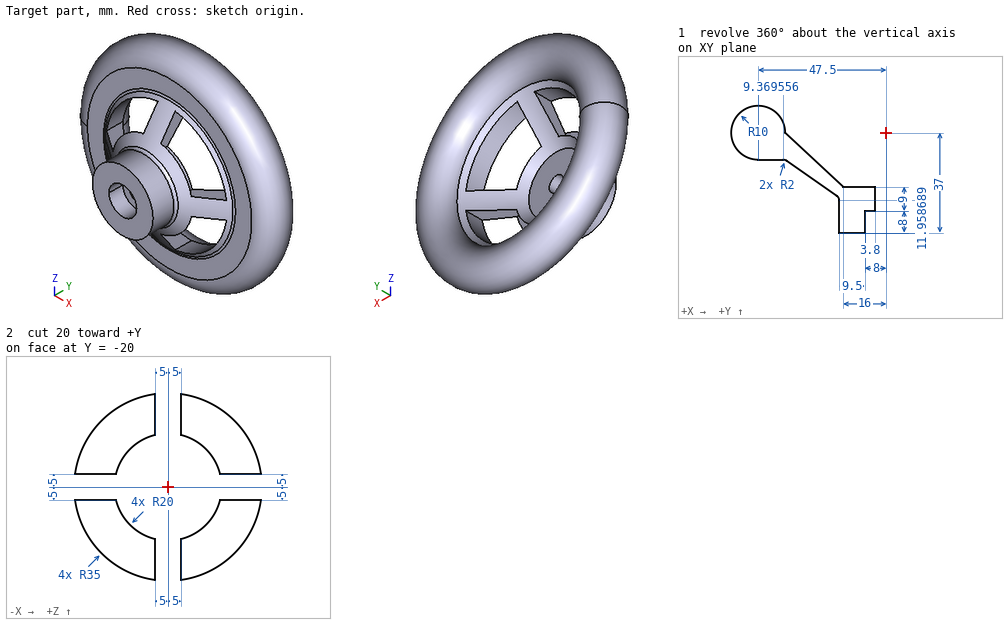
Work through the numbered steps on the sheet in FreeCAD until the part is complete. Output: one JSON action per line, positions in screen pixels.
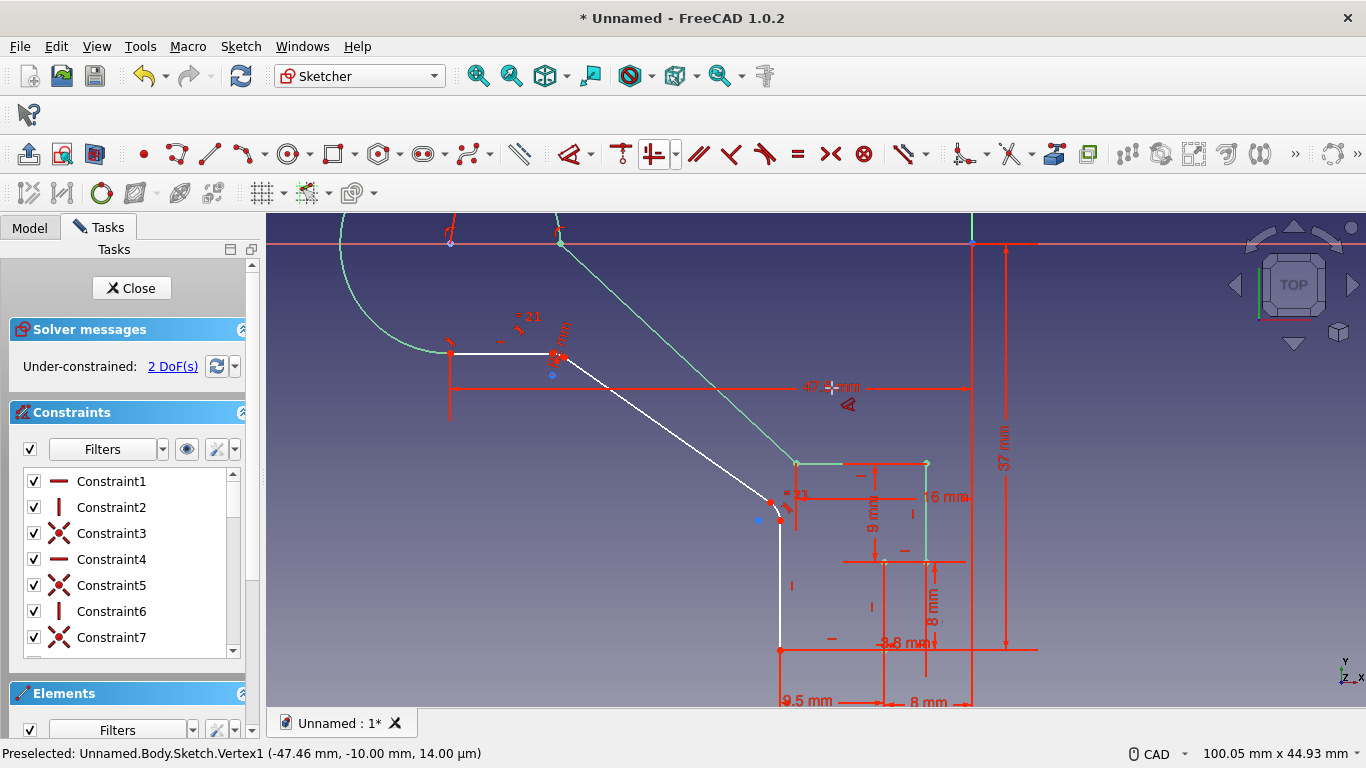
{"action": "left_click", "coordinate": [481, 354]}
{"action": "left_click", "coordinate": [501, 320]}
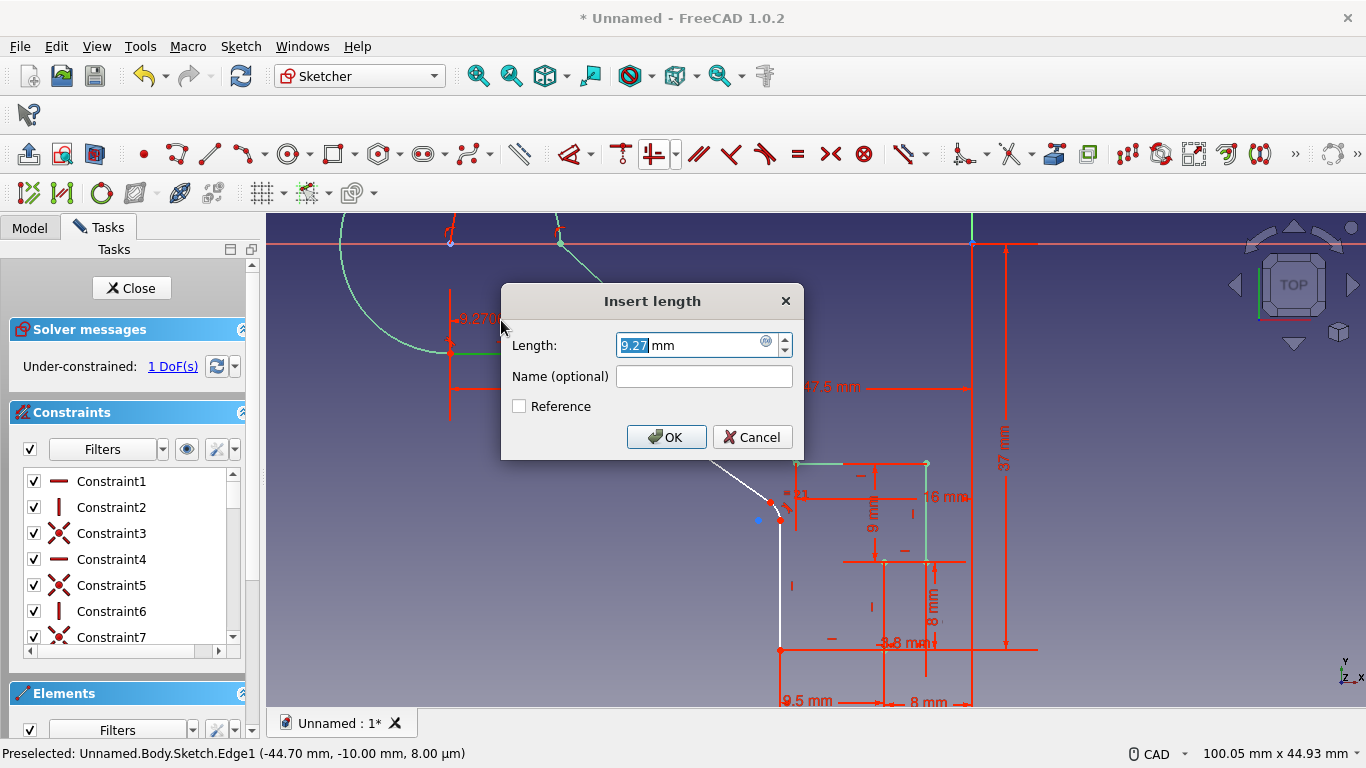
{"action": "type", "text": "9.369556"}
{"action": "key", "text": "Return"}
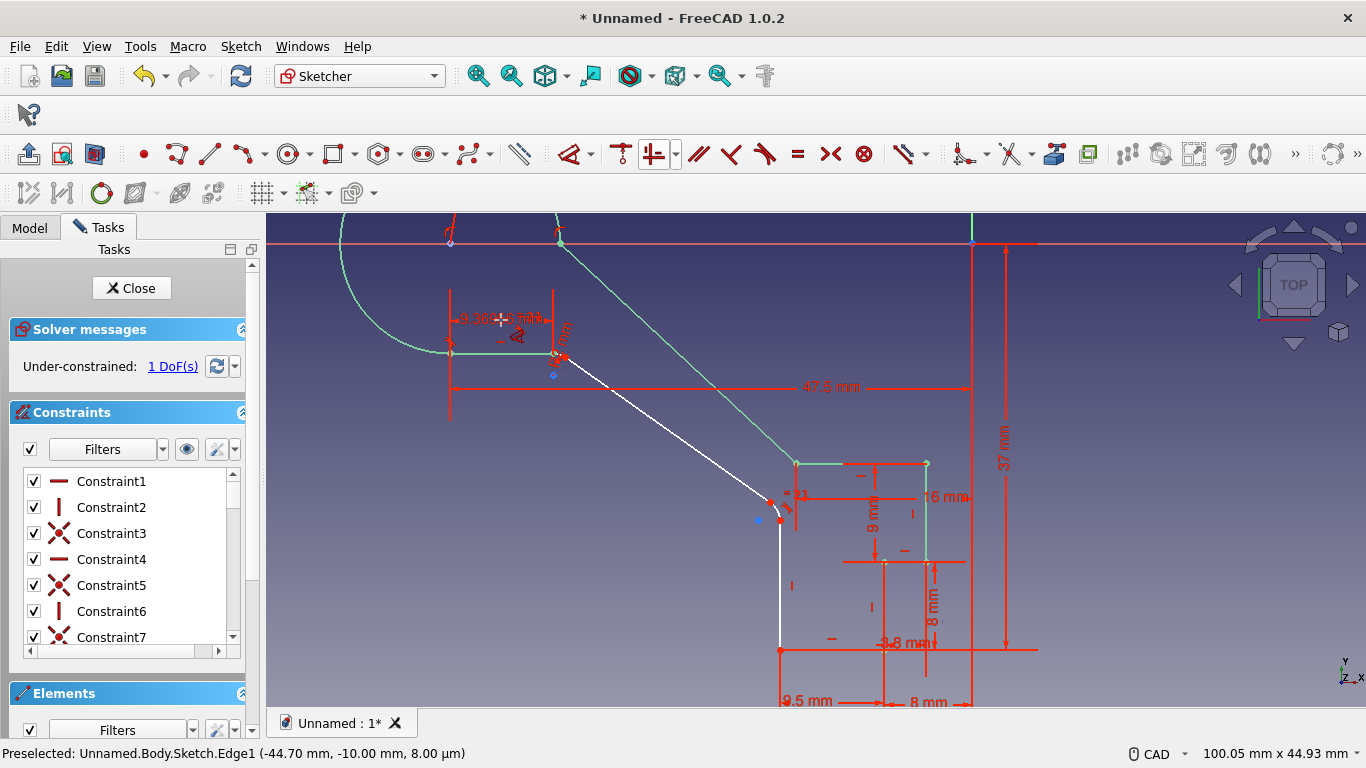
{"action": "left_click", "coordinate": [780, 560]}
{"action": "left_click", "coordinate": [814, 586]}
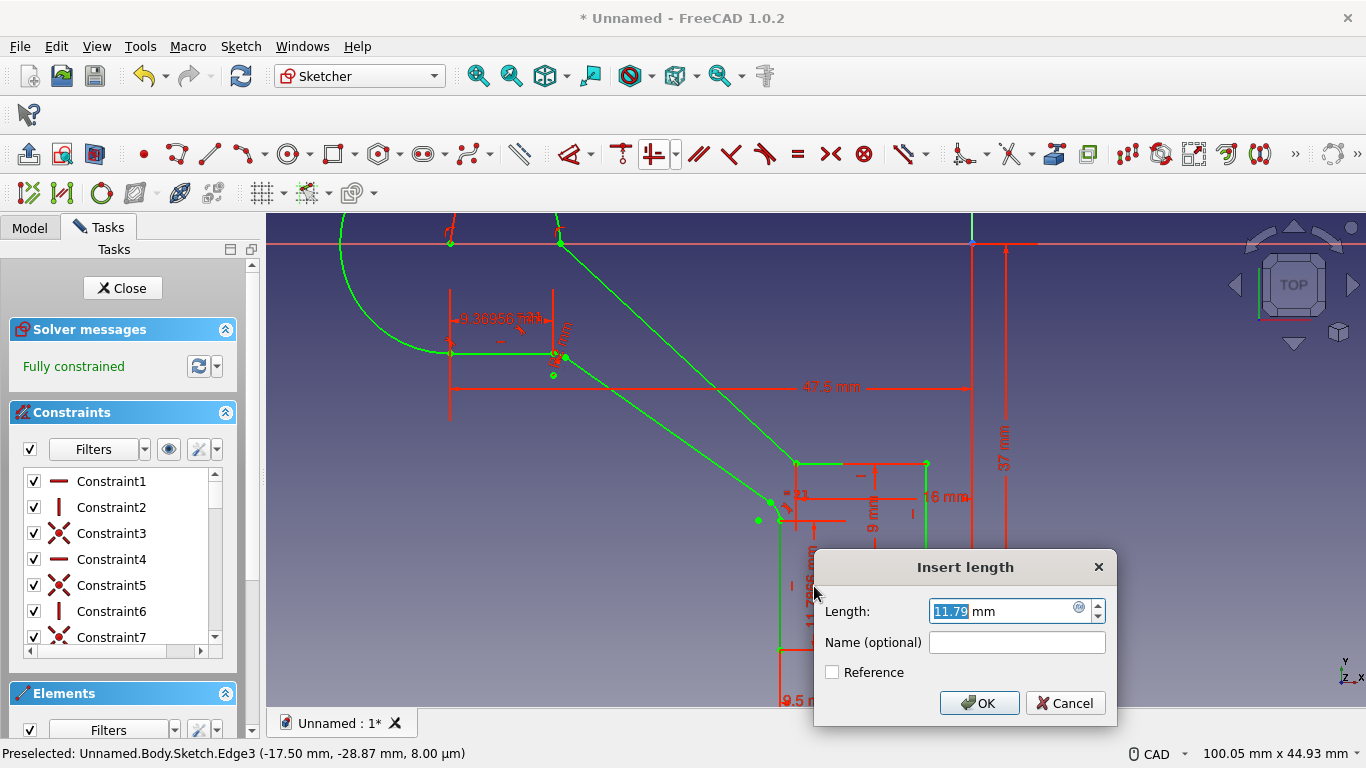
{"action": "type", "text": "11.958689"}
{"action": "key", "text": "Return"}
{"action": "key", "text": "Escape"}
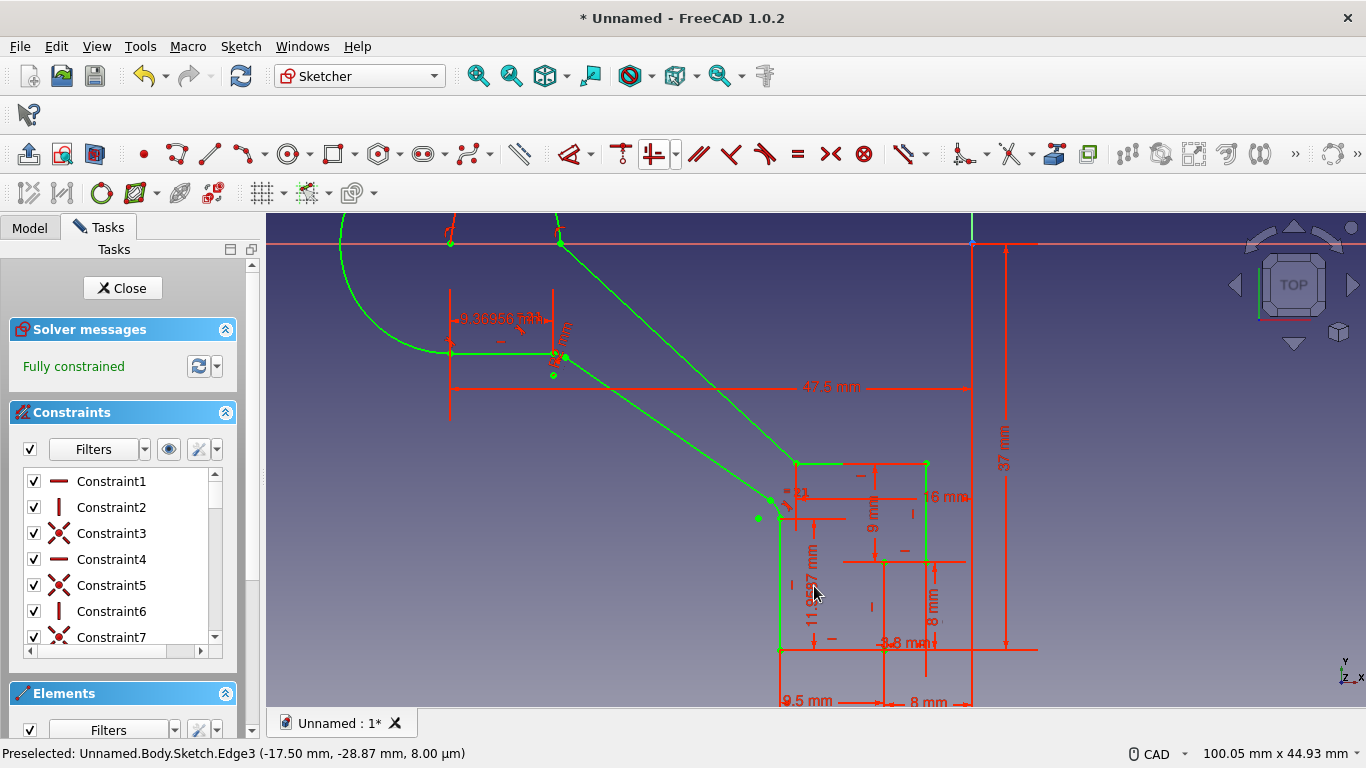
{"action": "left_click", "coordinate": [123, 288]}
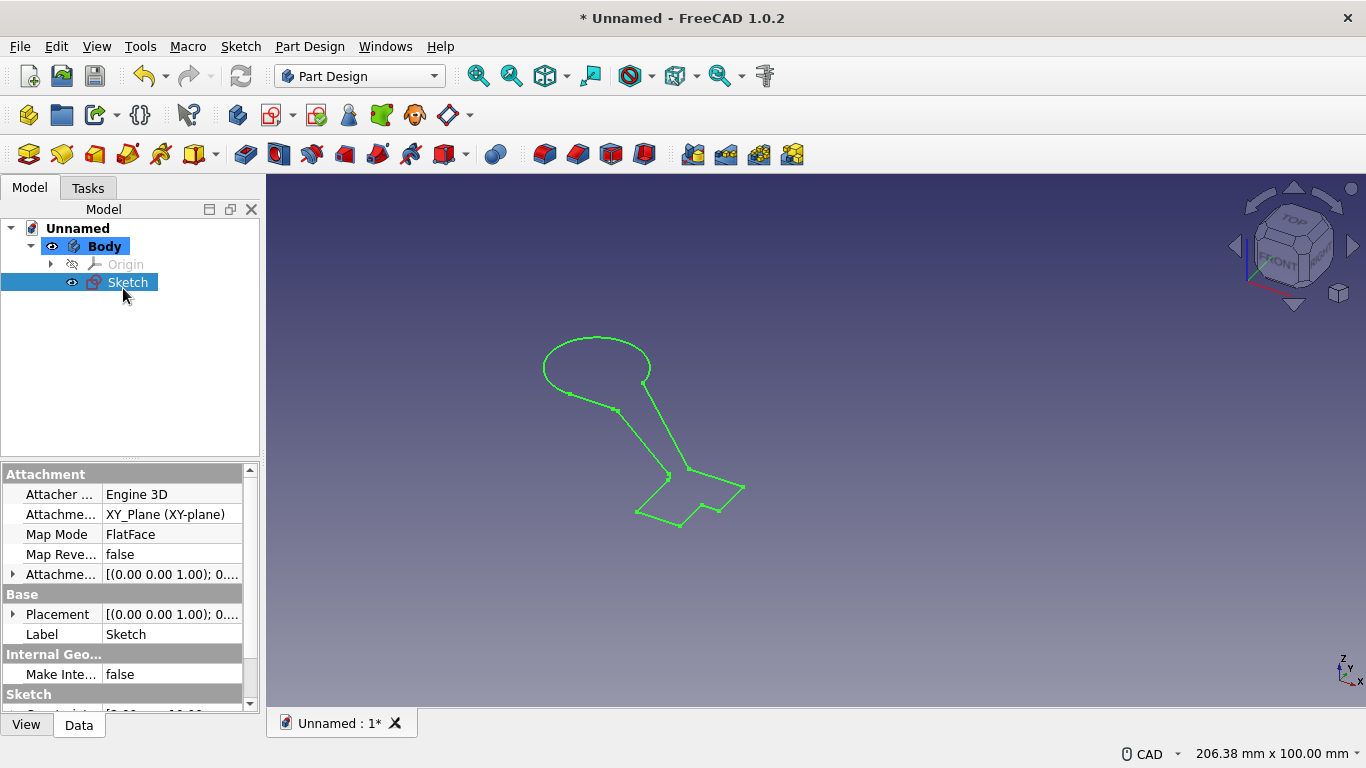
{"action": "left_click", "coordinate": [62, 154]}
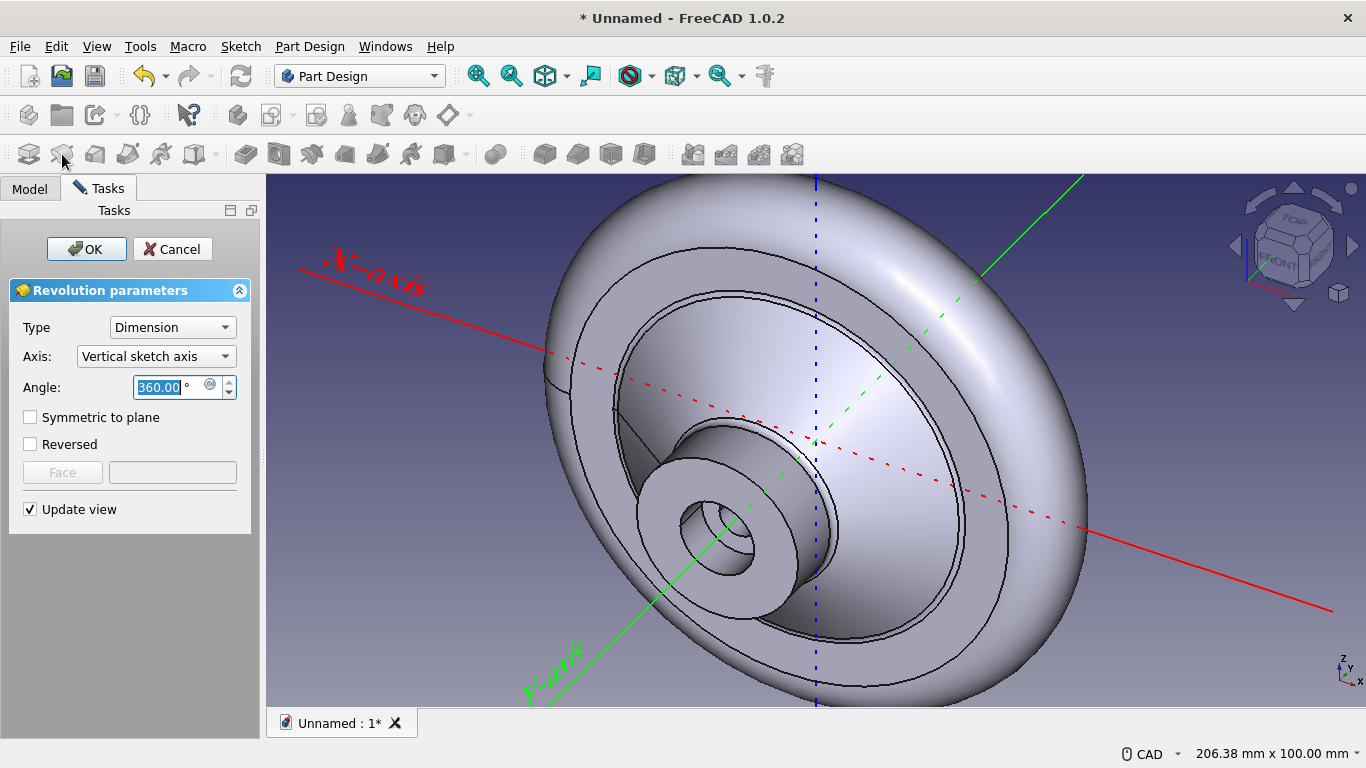
{"action": "left_click", "coordinate": [87, 249]}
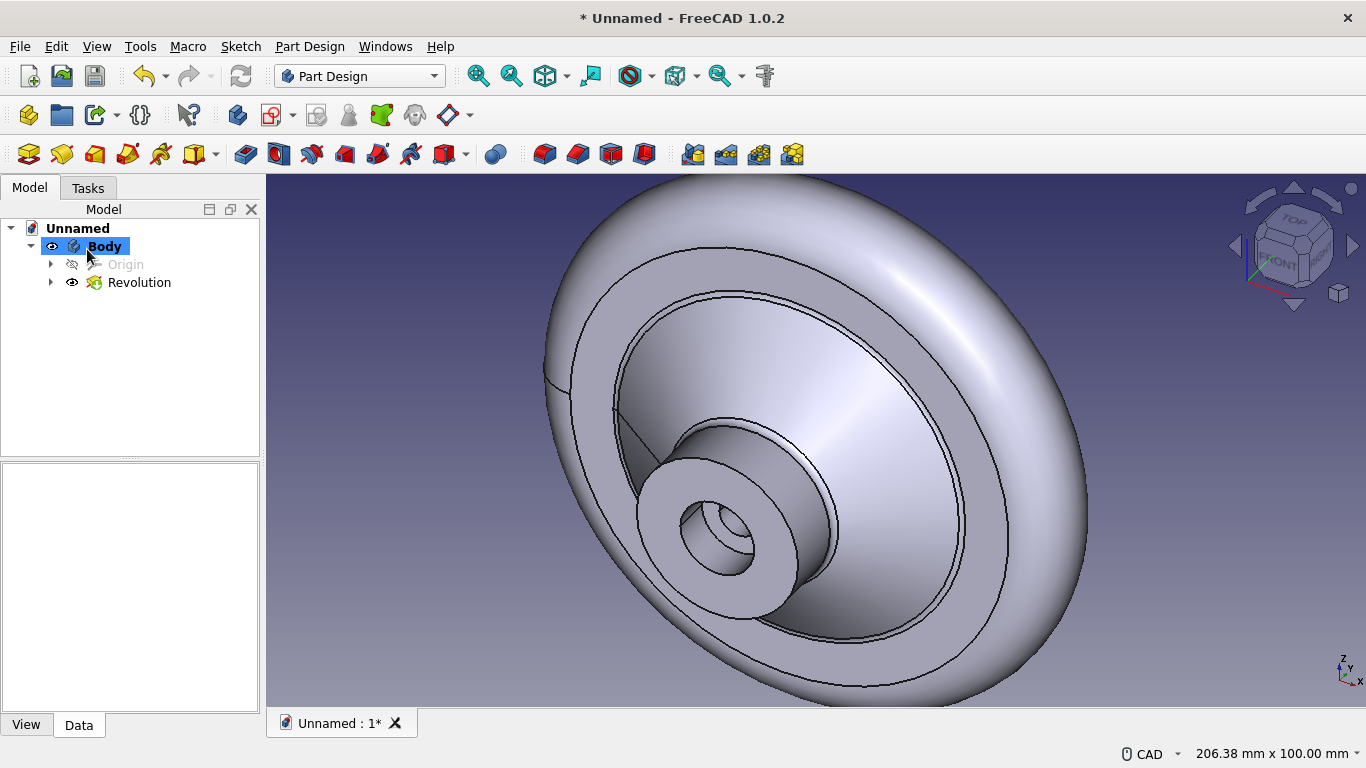
{"action": "key", "text": "v f"}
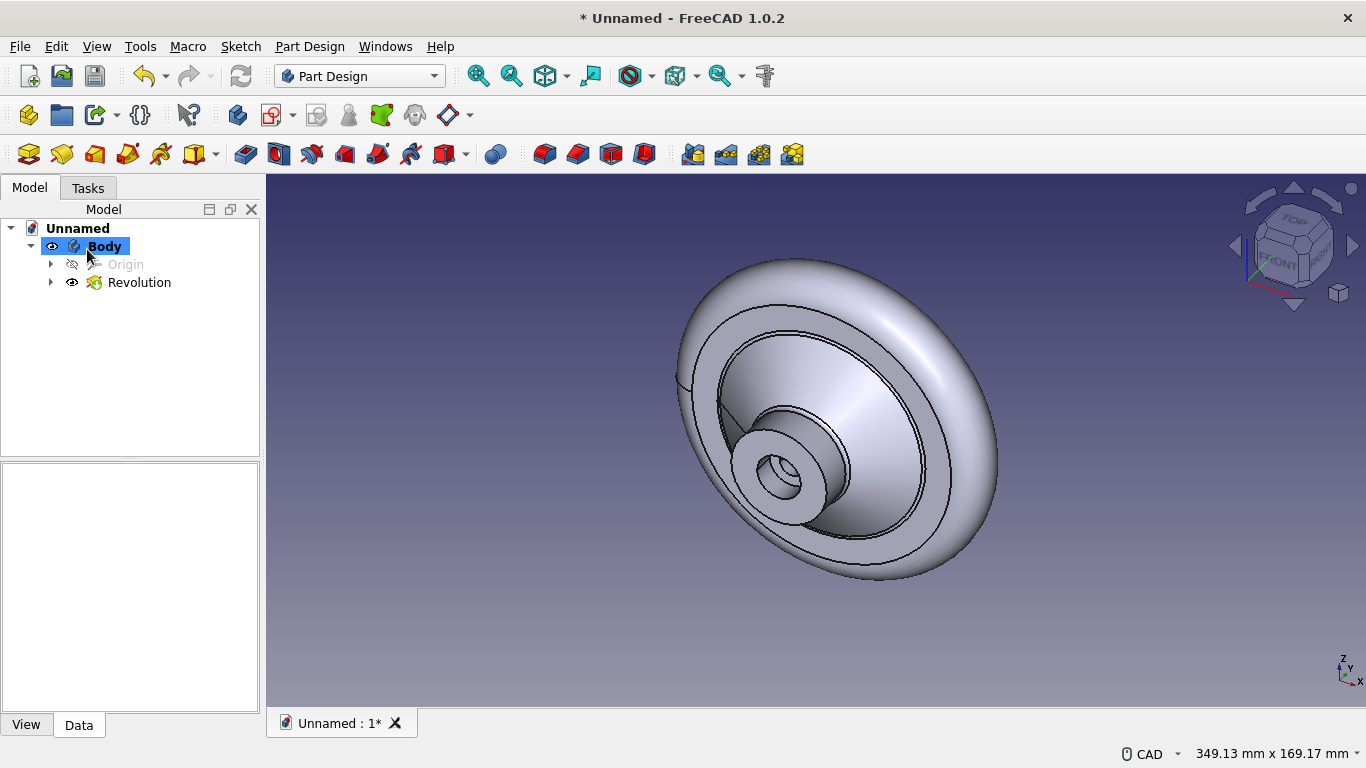
{"action": "key", "text": "4"}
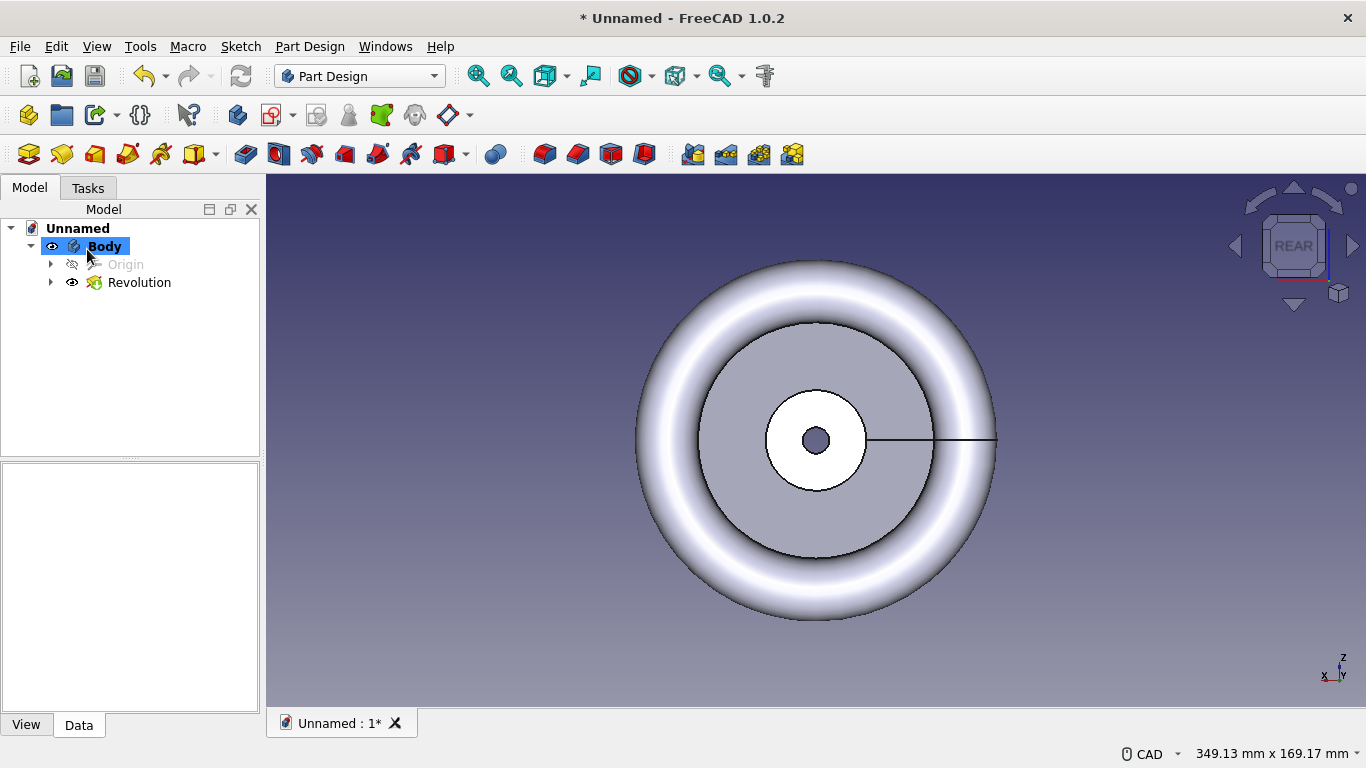
{"action": "left_click", "coordinate": [787, 454]}